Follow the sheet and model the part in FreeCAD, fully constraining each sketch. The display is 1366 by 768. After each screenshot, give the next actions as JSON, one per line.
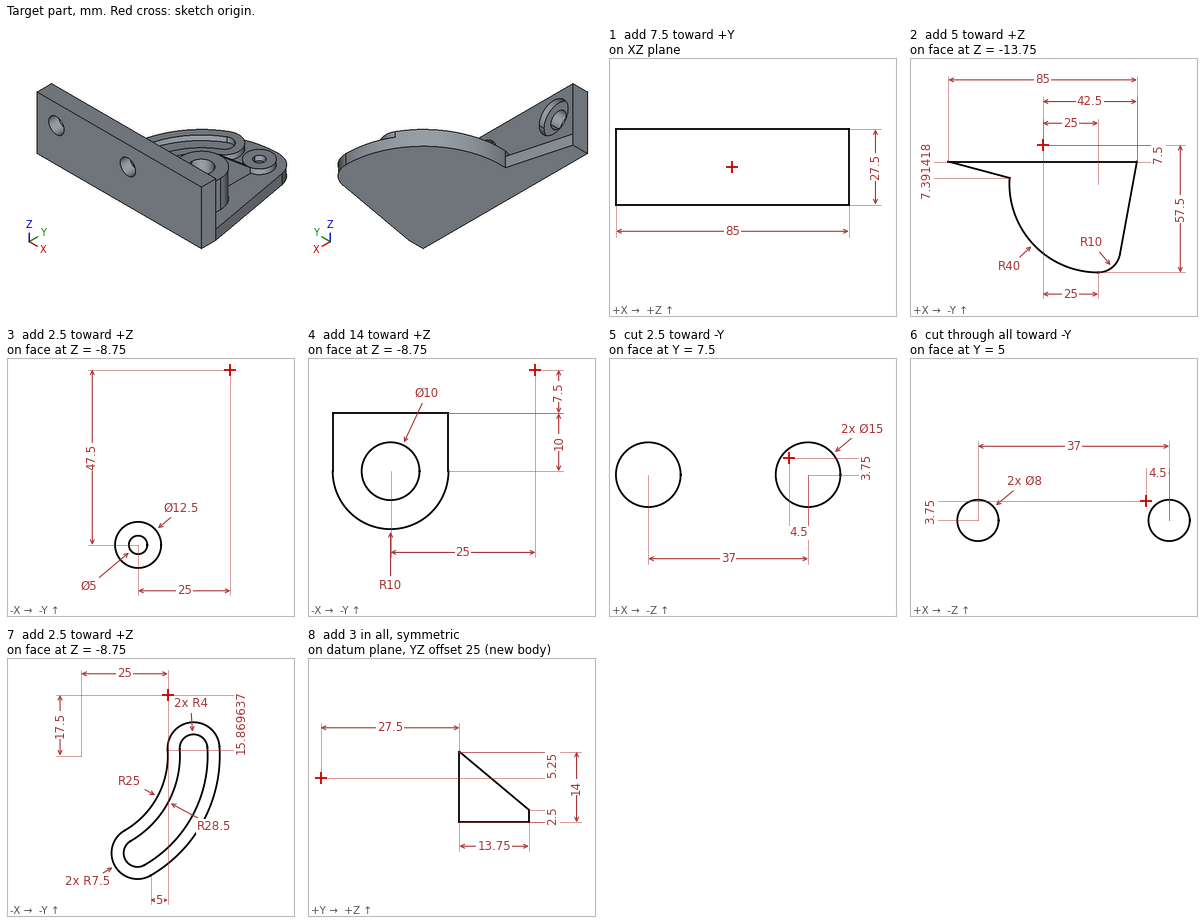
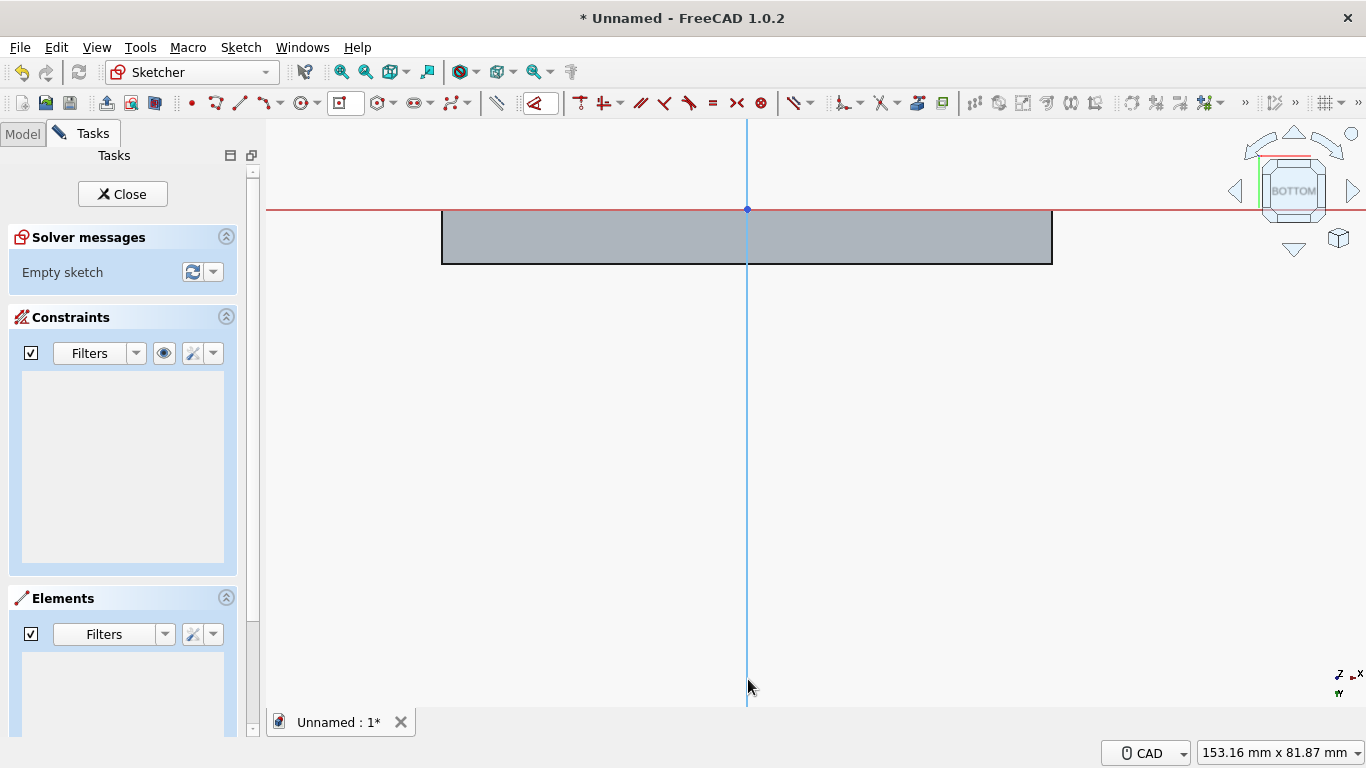
{"action": "left_click", "coordinate": [216, 104]}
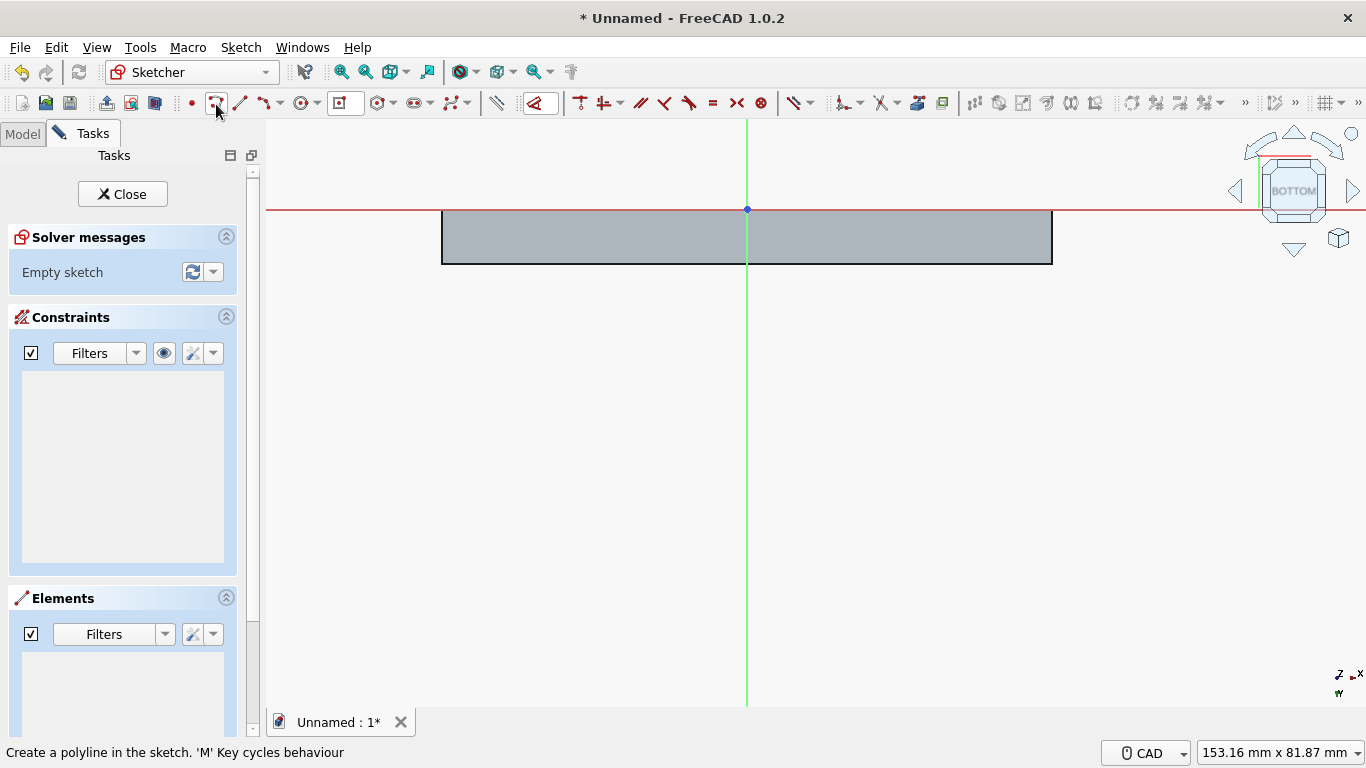
{"action": "left_click", "coordinate": [997, 564]}
{"action": "left_click", "coordinate": [1052, 264]}
{"action": "left_click", "coordinate": [442, 264]}
{"action": "left_click", "coordinate": [640, 317]}
{"action": "right_click", "coordinate": [640, 317]}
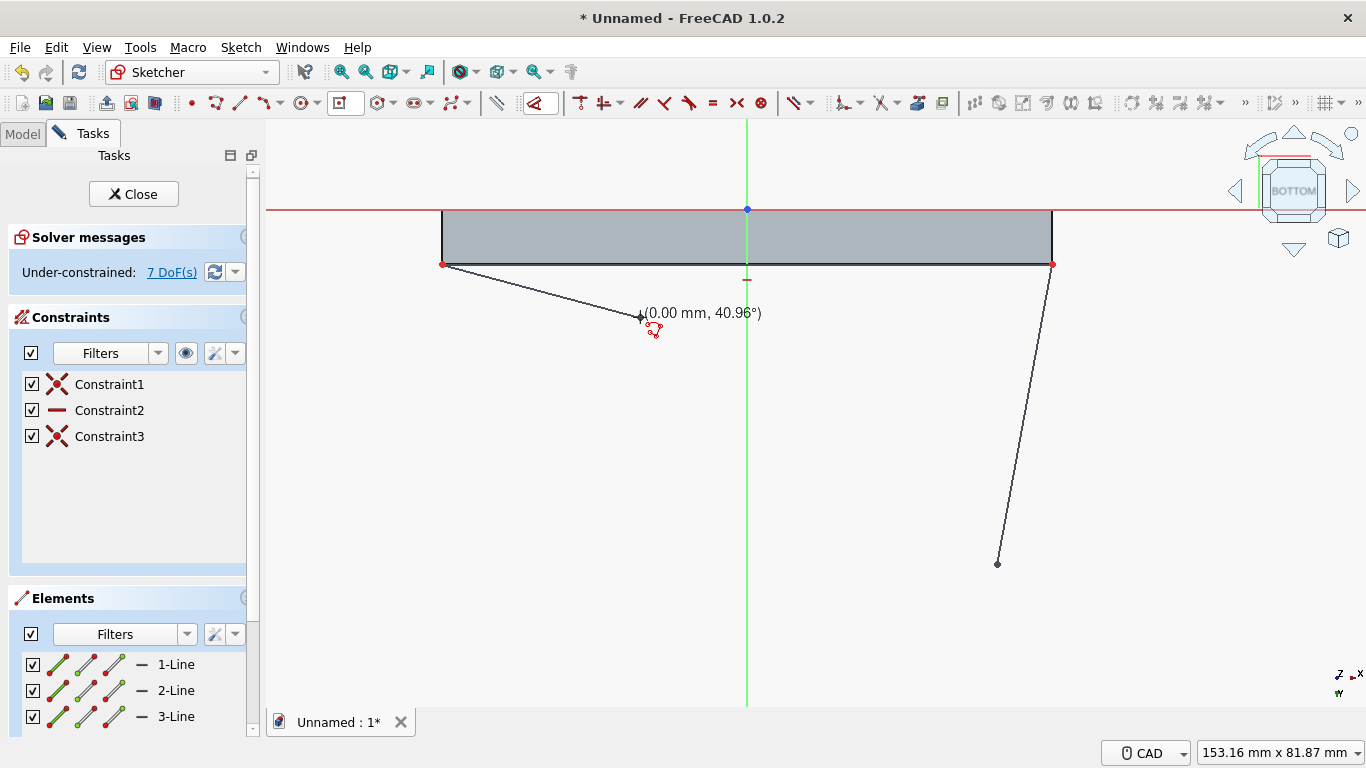
{"action": "left_click", "coordinate": [264, 104]}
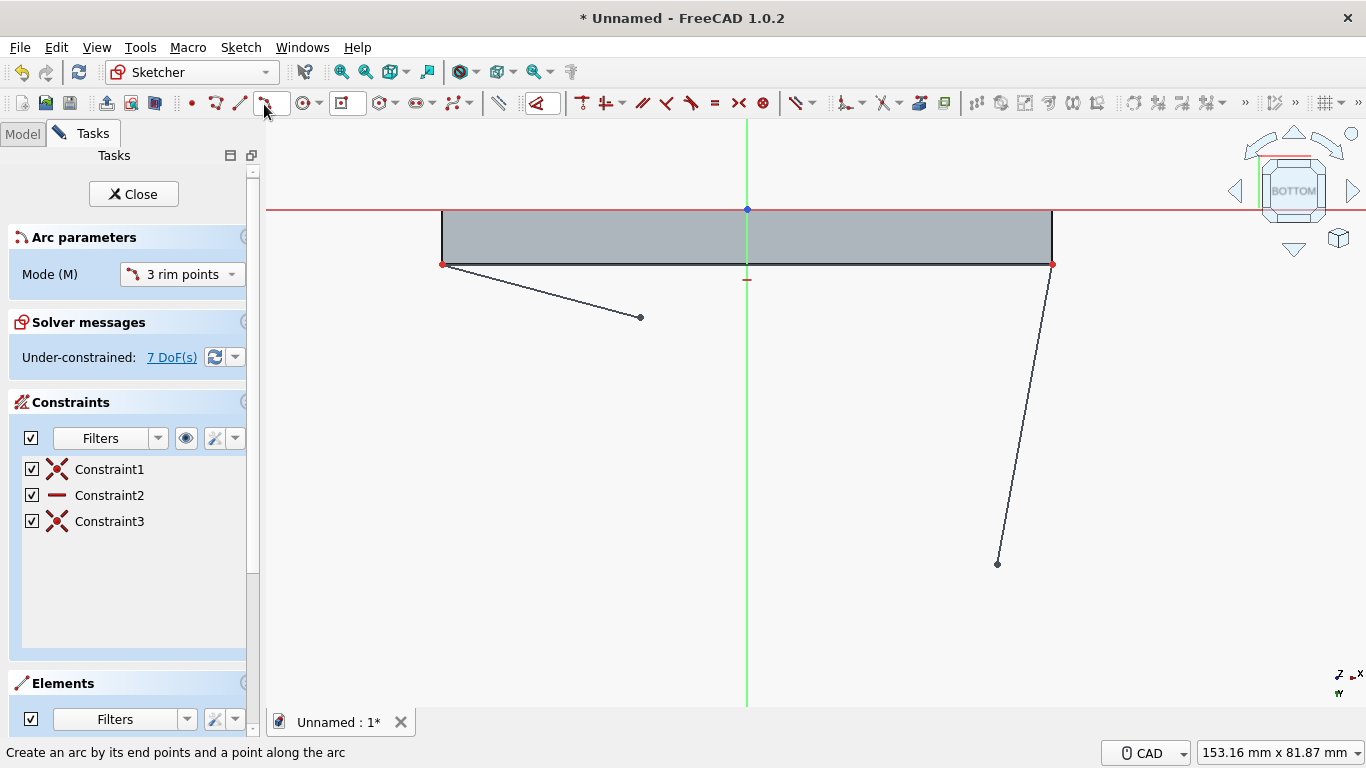
{"action": "left_click", "coordinate": [640, 318]}
{"action": "left_click", "coordinate": [927, 623]}
{"action": "left_click", "coordinate": [717, 532]}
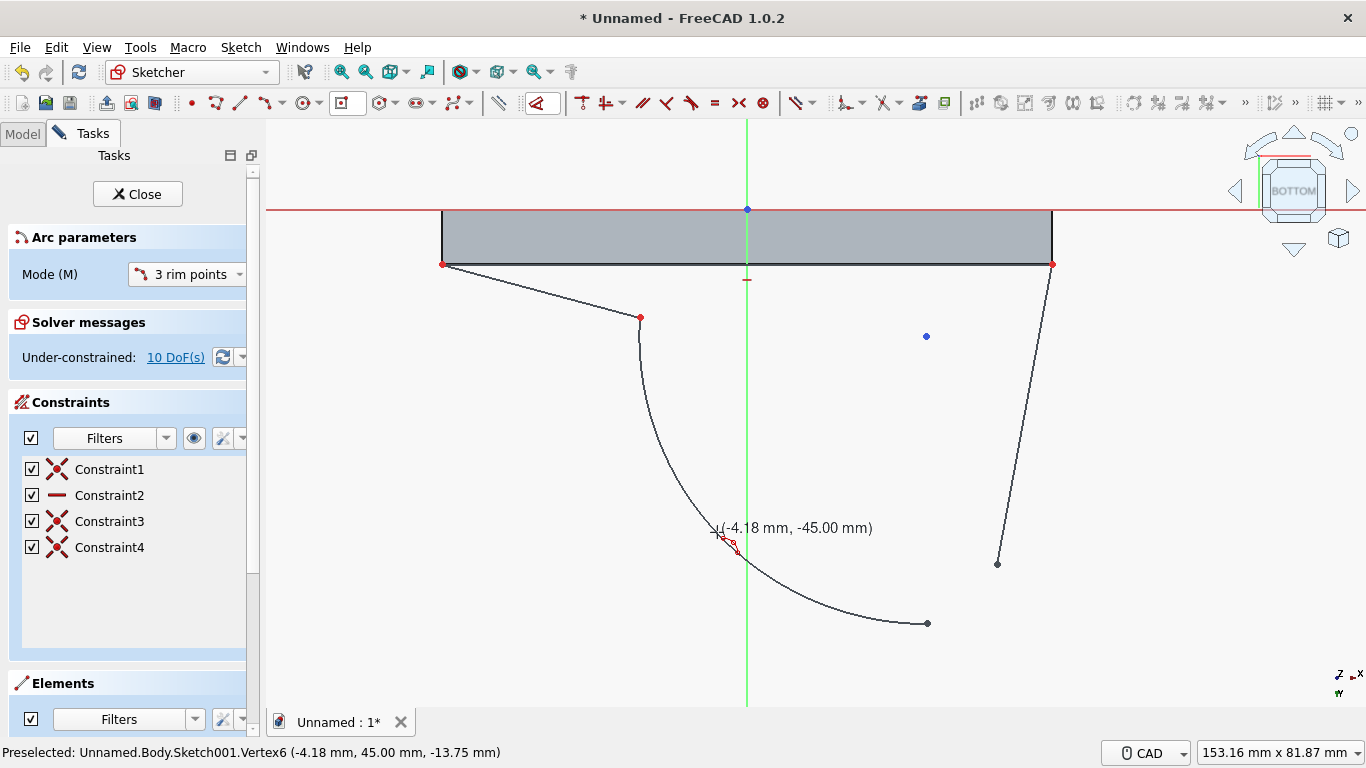
{"action": "left_click", "coordinate": [927, 624]}
{"action": "left_click", "coordinate": [997, 565]}
{"action": "left_click", "coordinate": [973, 606]}
{"action": "key", "text": "Escape"}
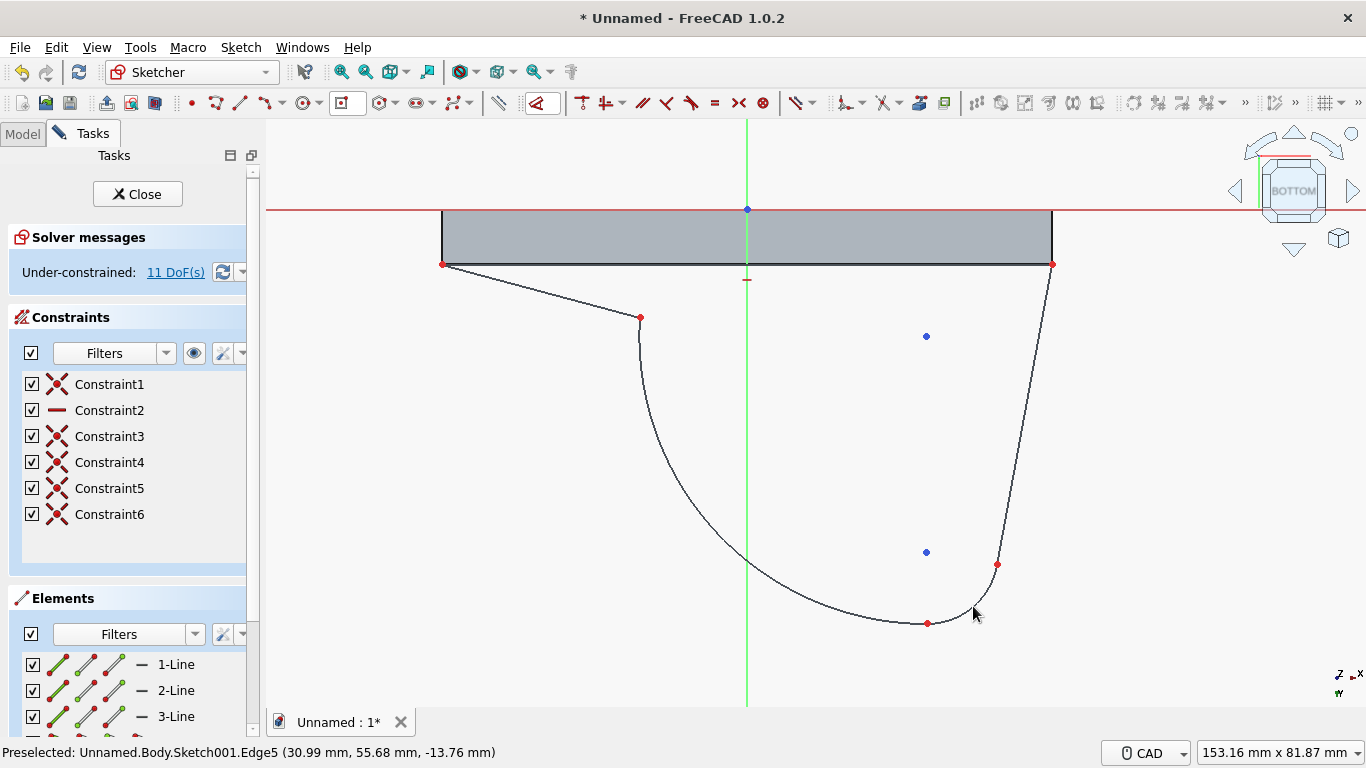
{"action": "left_click", "coordinate": [1014, 475]}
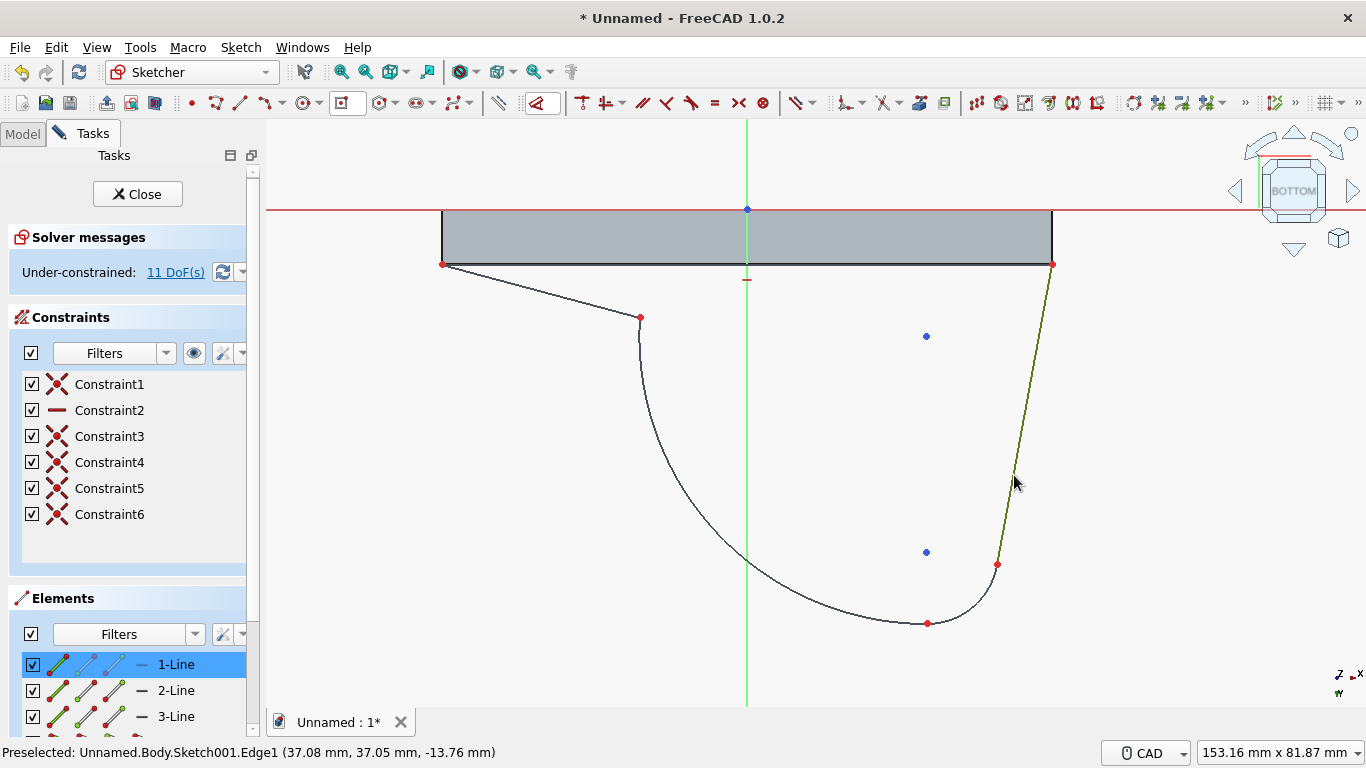
{"action": "left_click", "coordinate": [956, 618]}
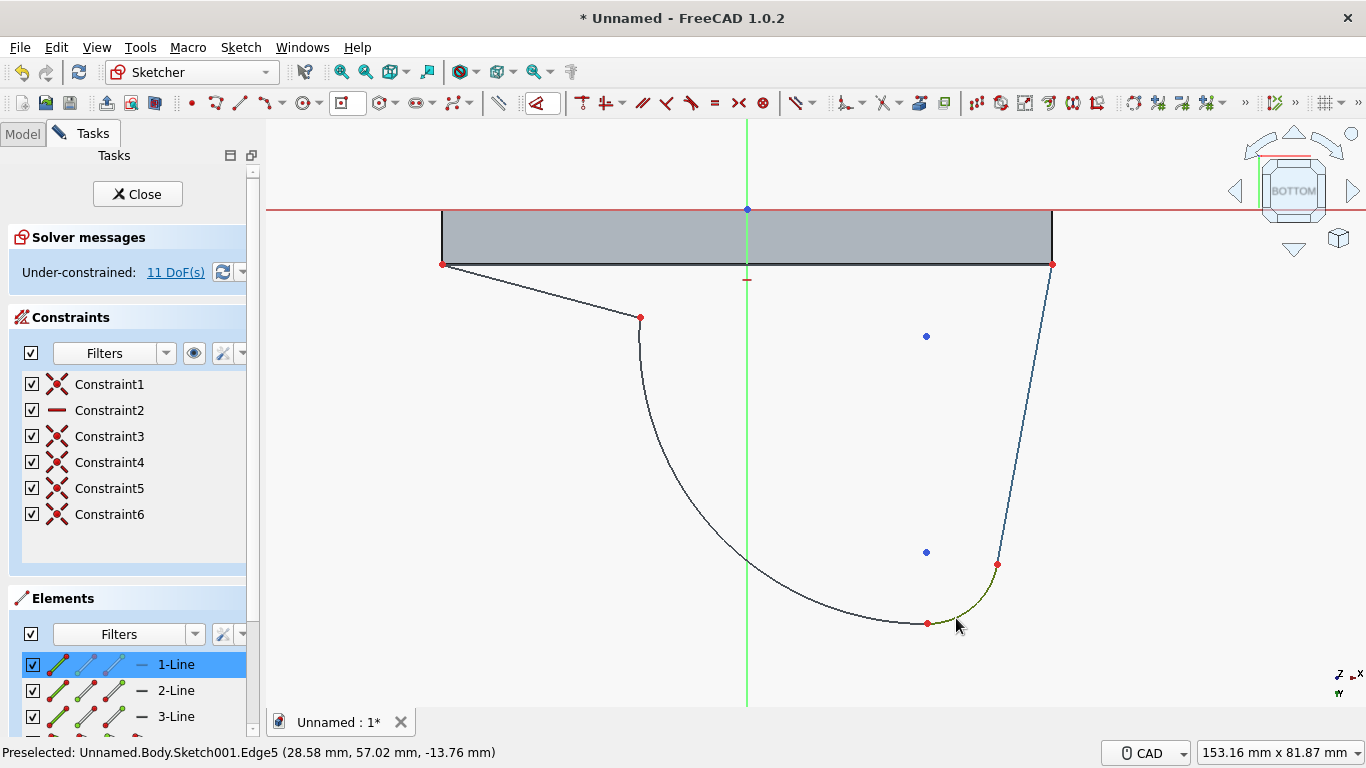
{"action": "left_click", "coordinate": [692, 104]}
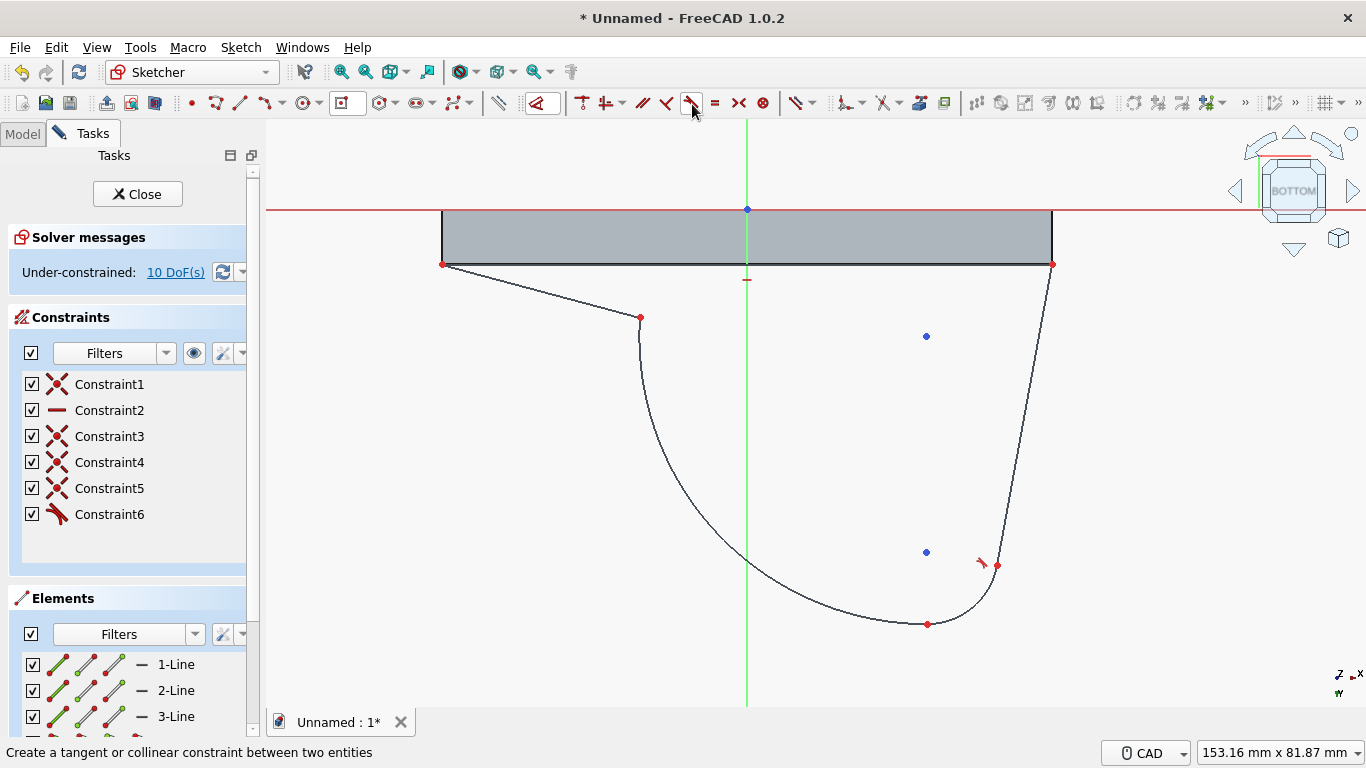
{"action": "left_click", "coordinate": [665, 455]}